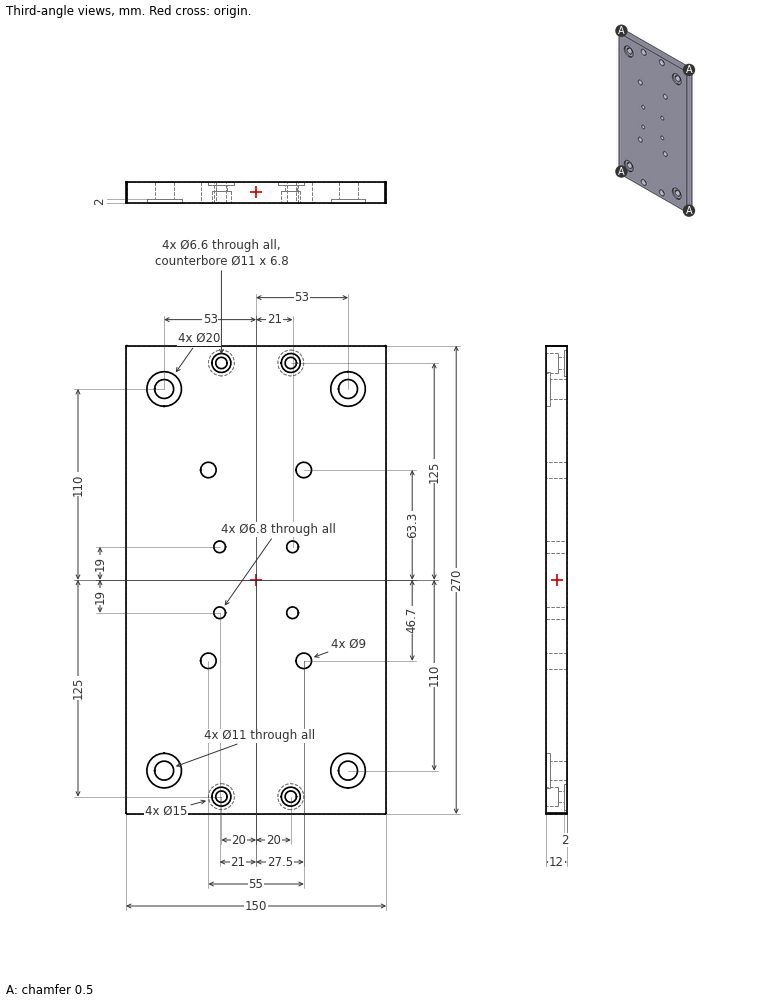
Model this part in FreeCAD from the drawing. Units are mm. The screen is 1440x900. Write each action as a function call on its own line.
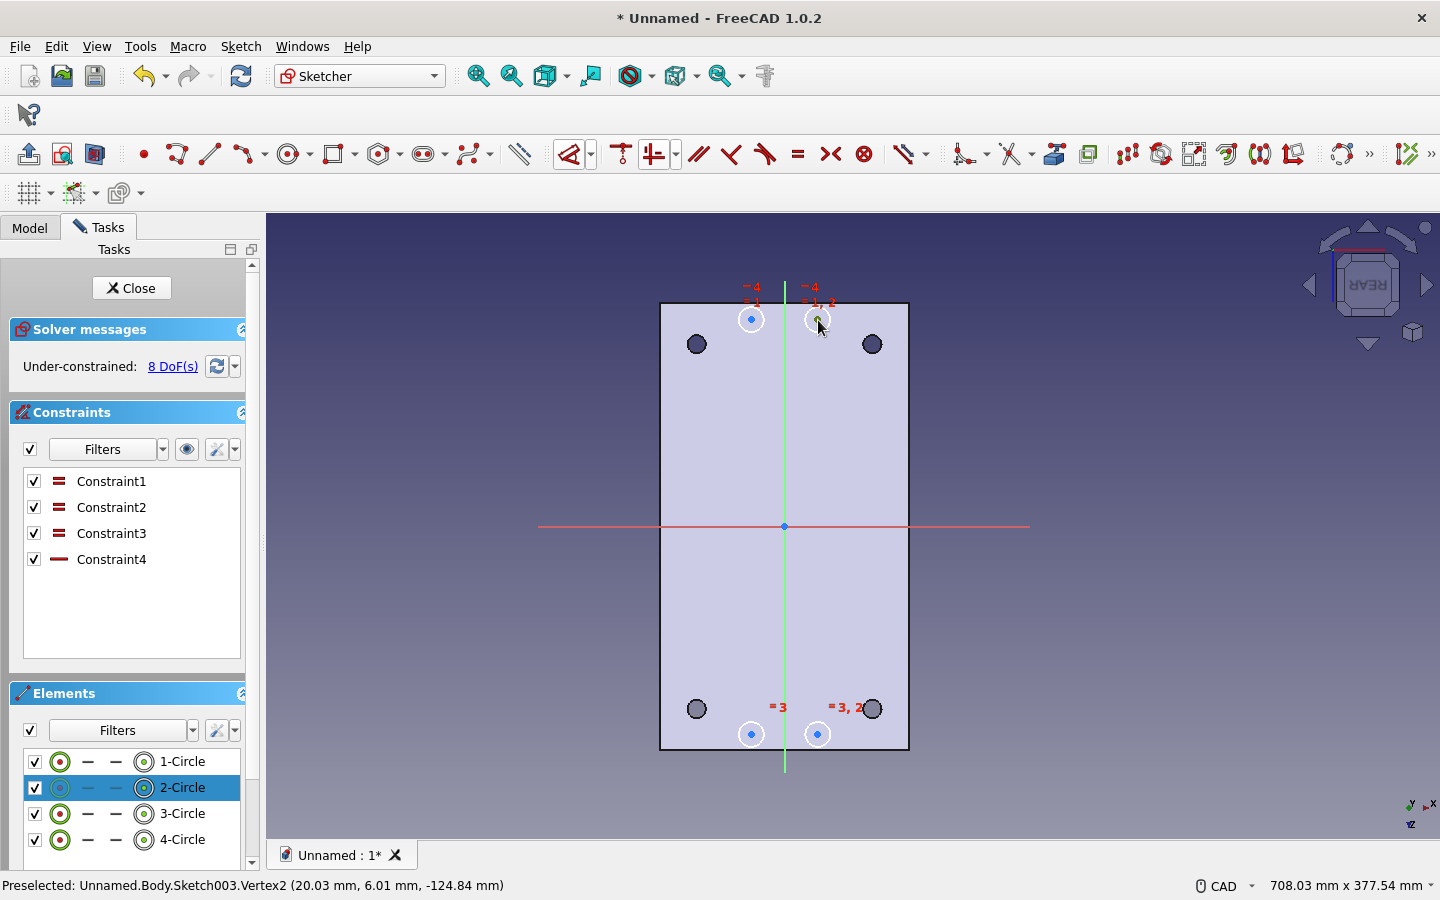
click(818, 734)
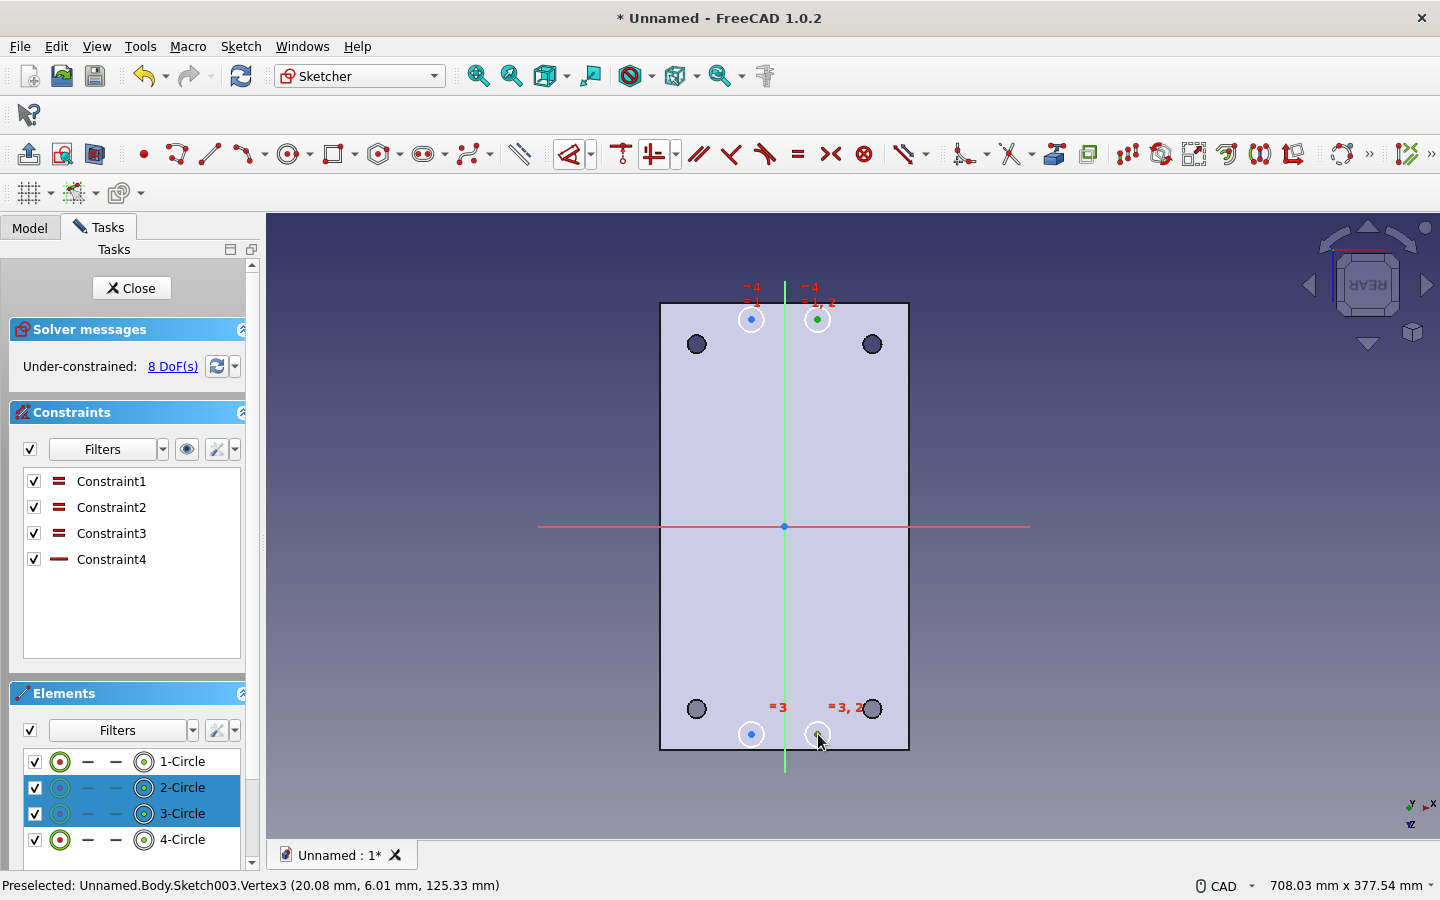
key(v)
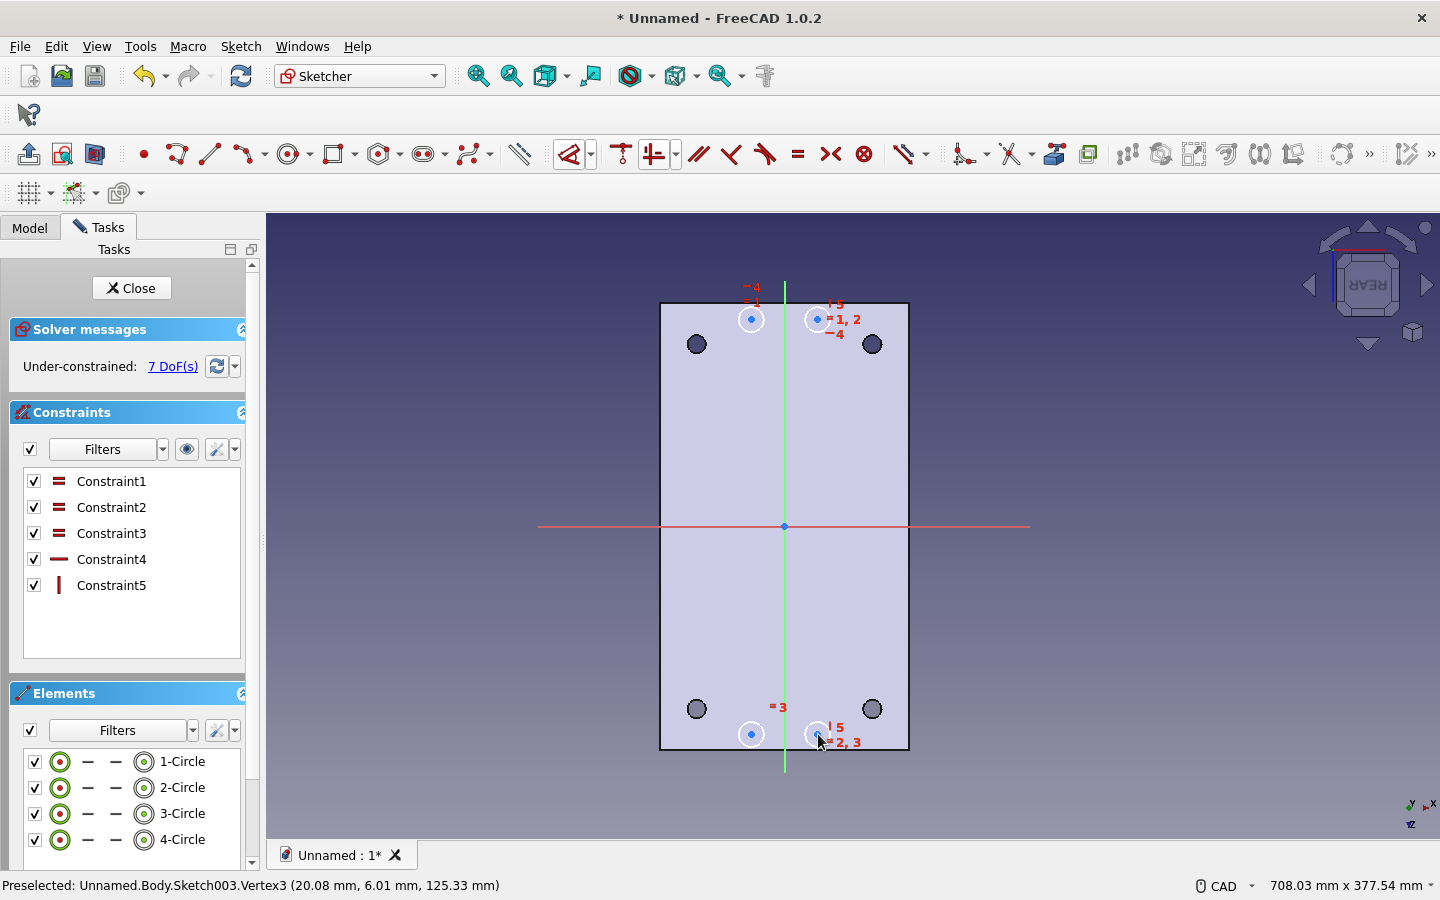
click(751, 320)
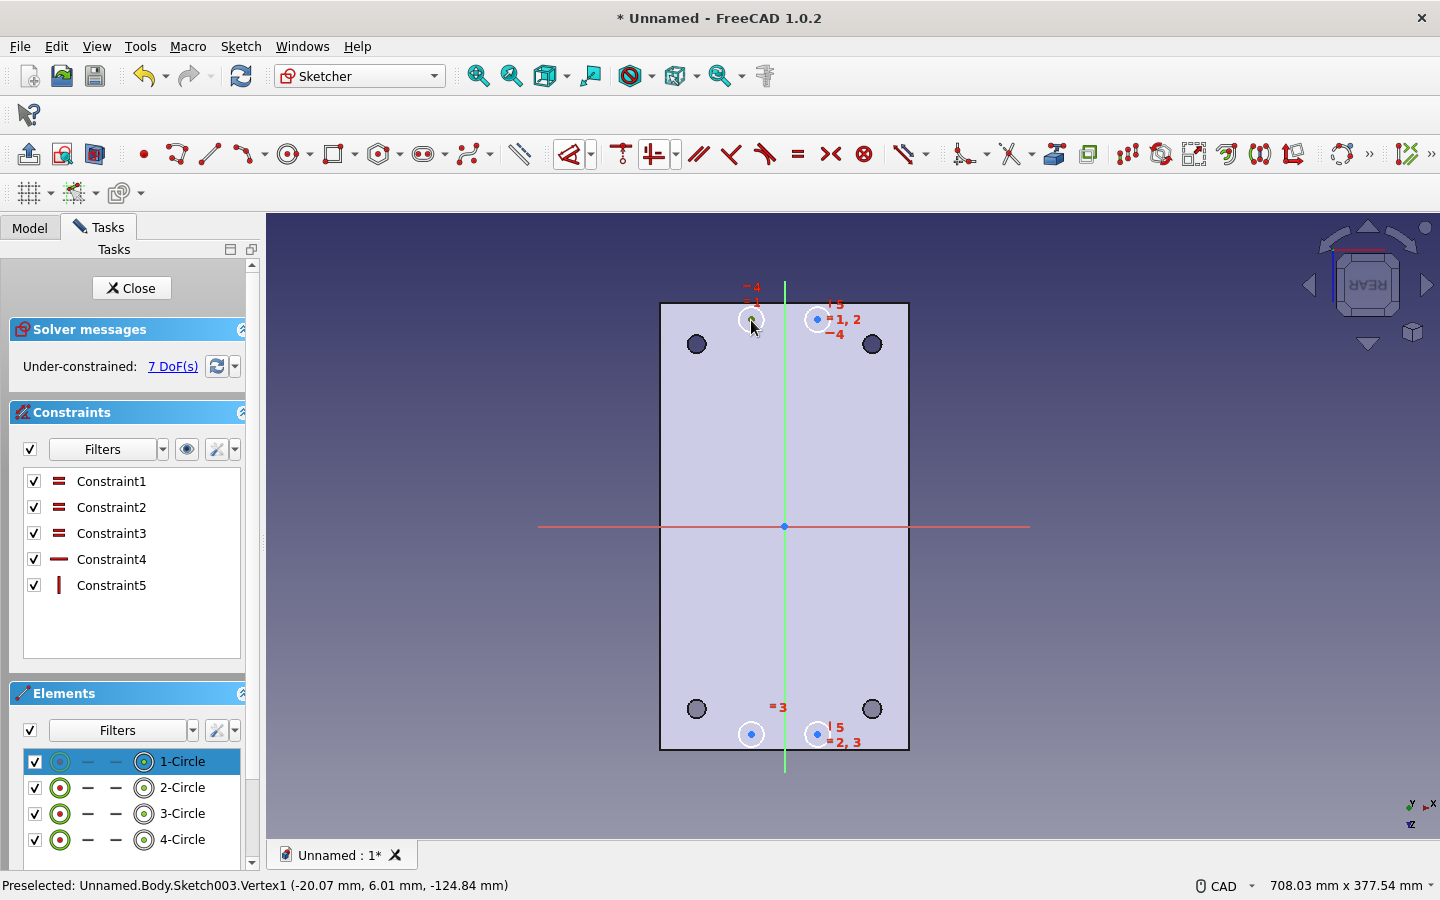
click(751, 734)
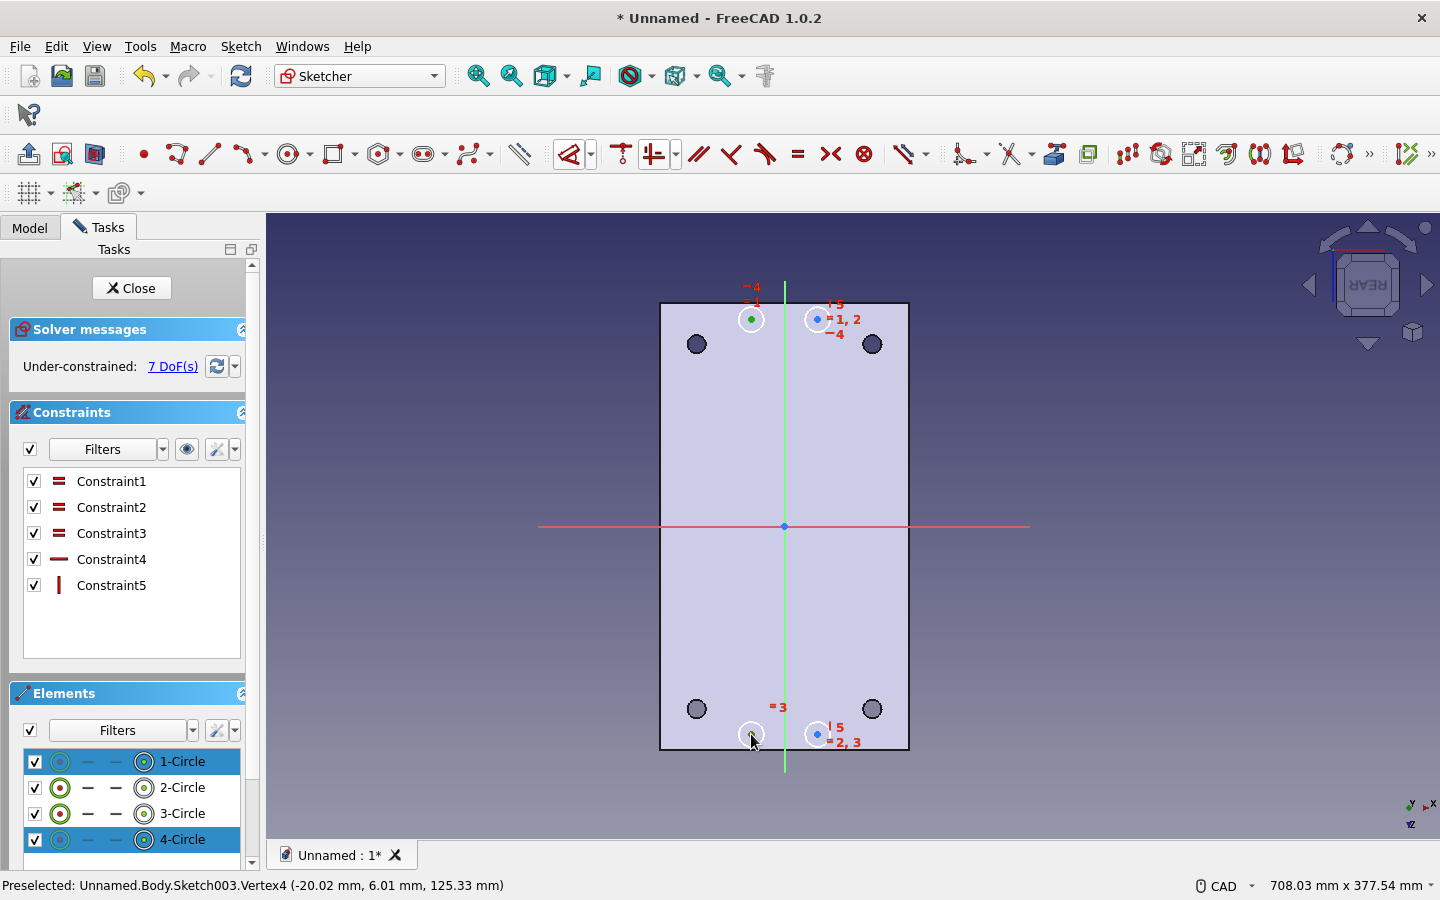
click(676, 154)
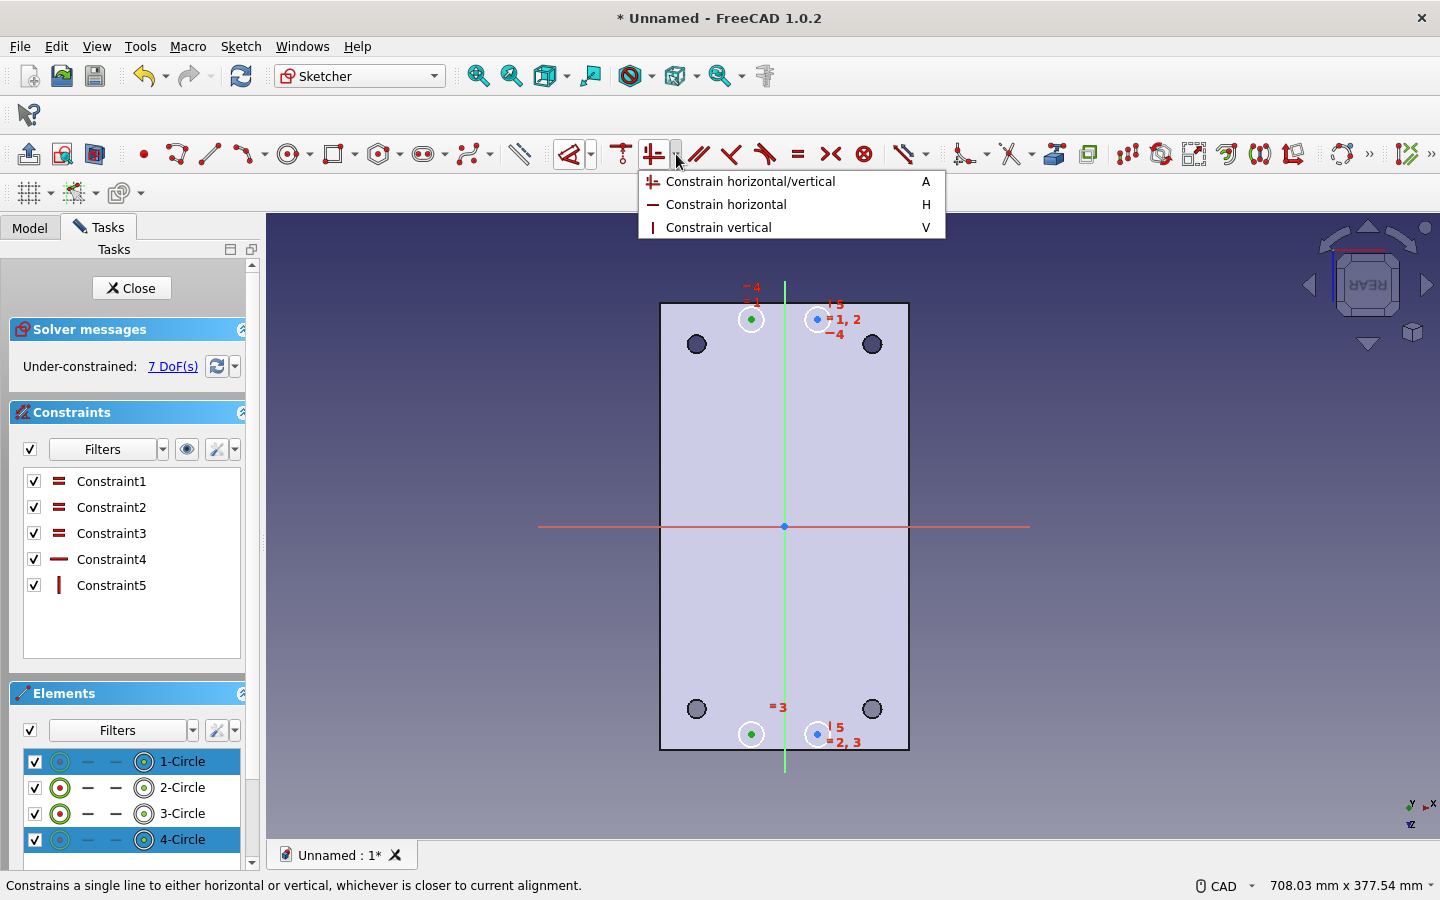
click(792, 228)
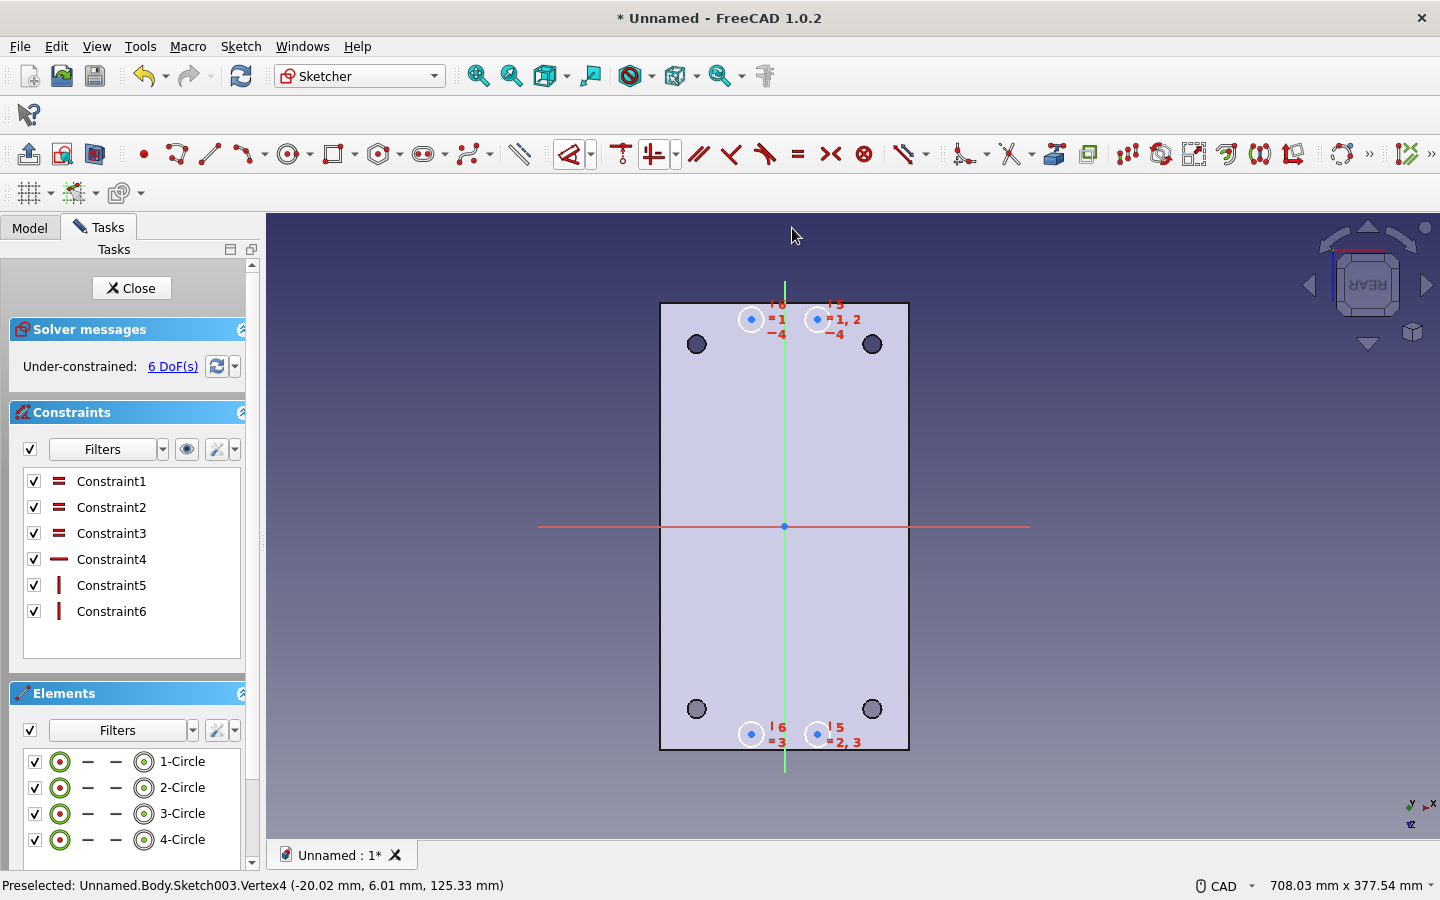
click(818, 734)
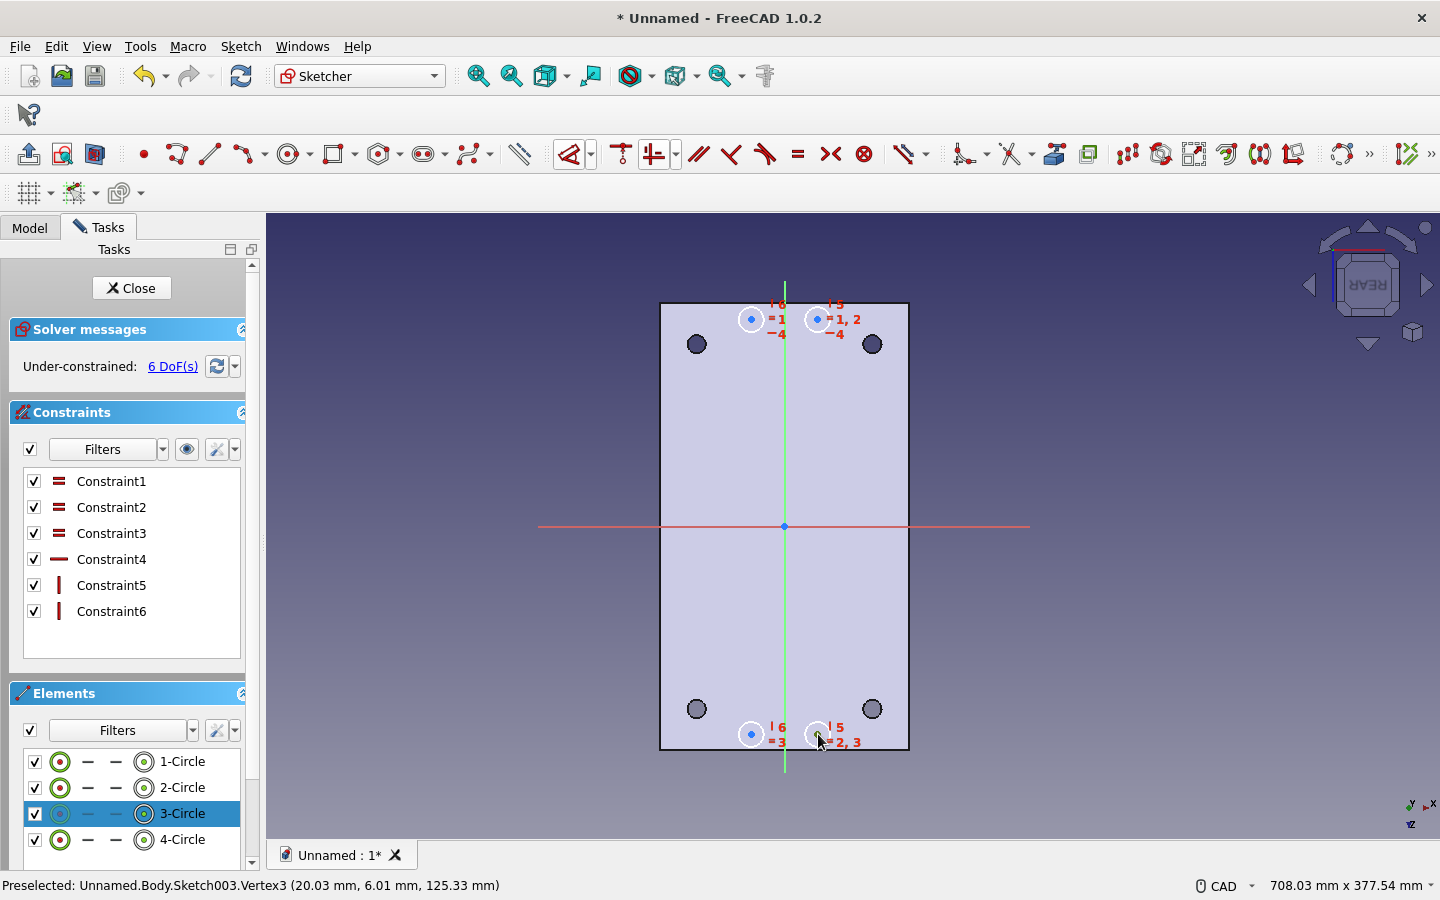
click(751, 734)